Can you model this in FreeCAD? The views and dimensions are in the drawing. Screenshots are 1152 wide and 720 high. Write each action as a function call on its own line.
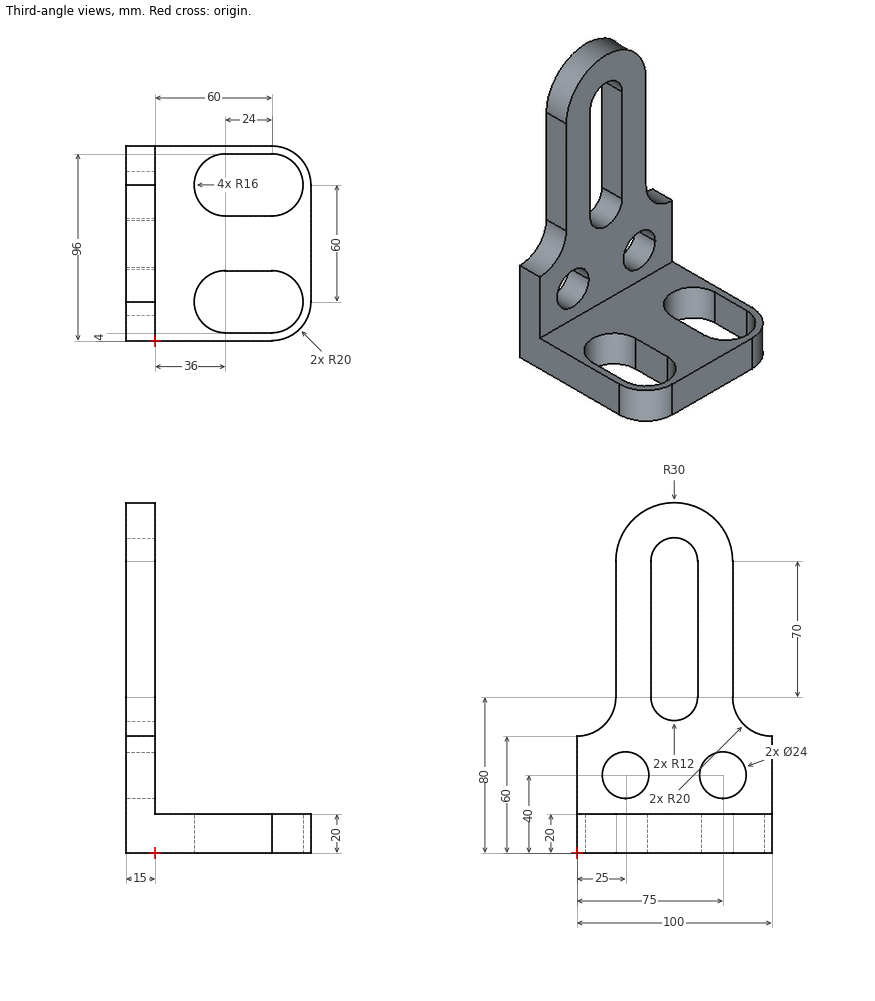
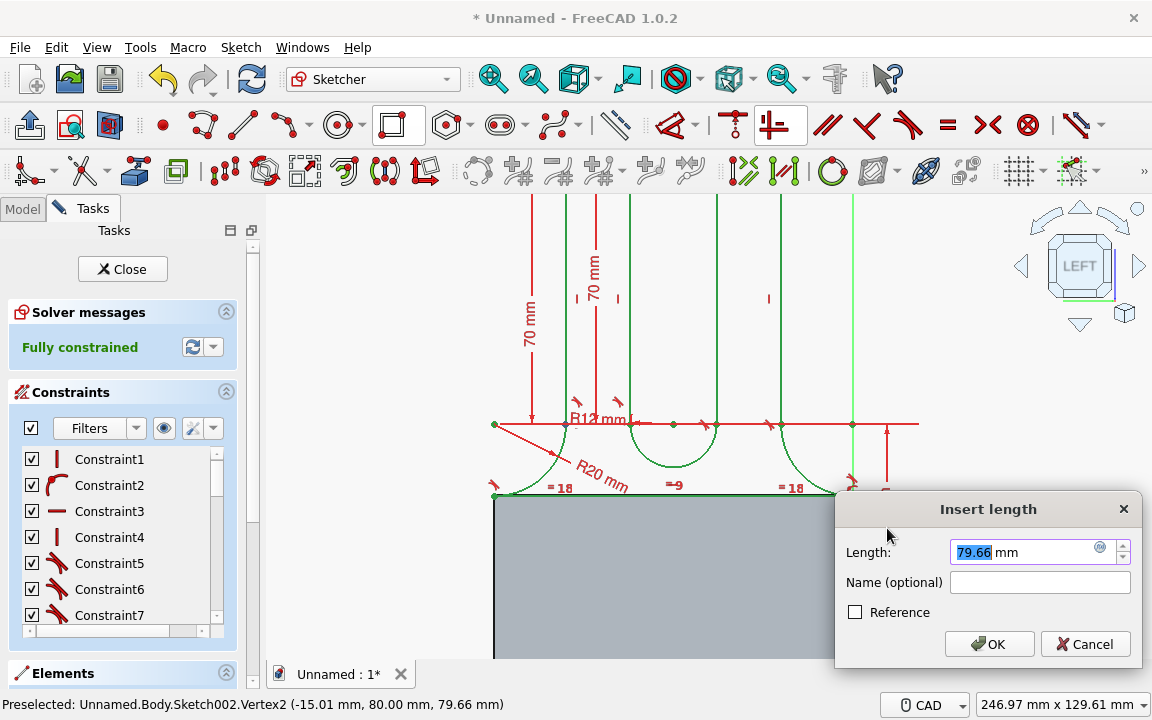
text(80)
key(Return)
key(Escape)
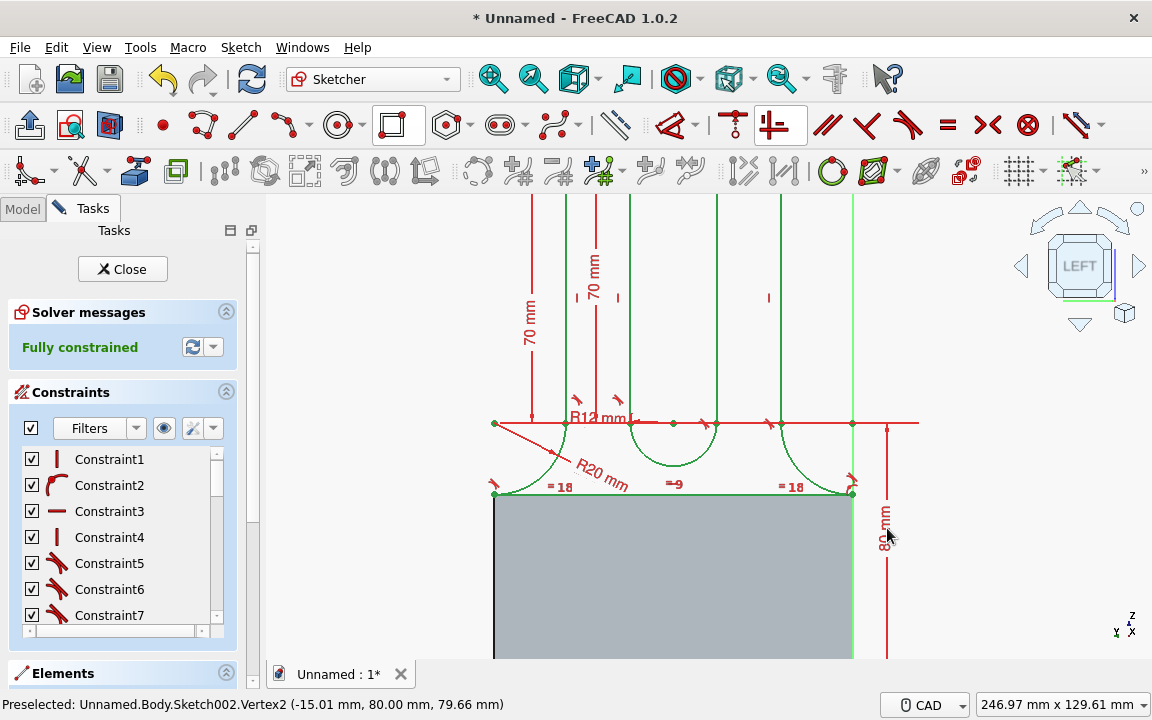
click(123, 269)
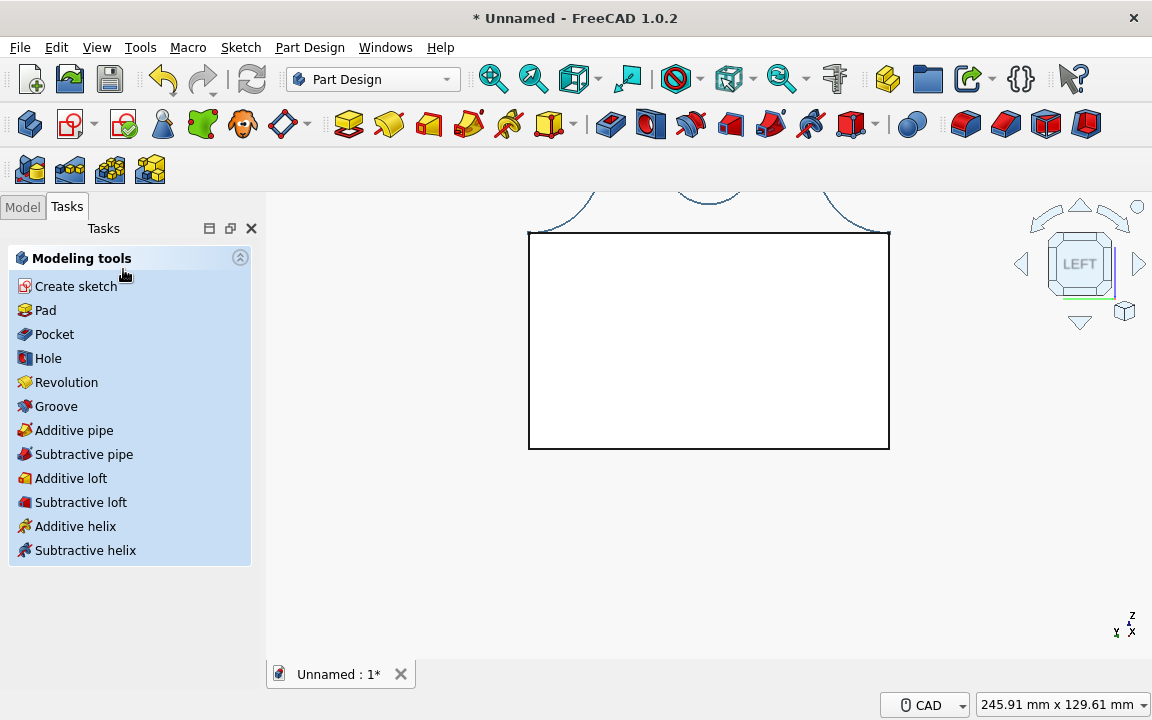
click(350, 124)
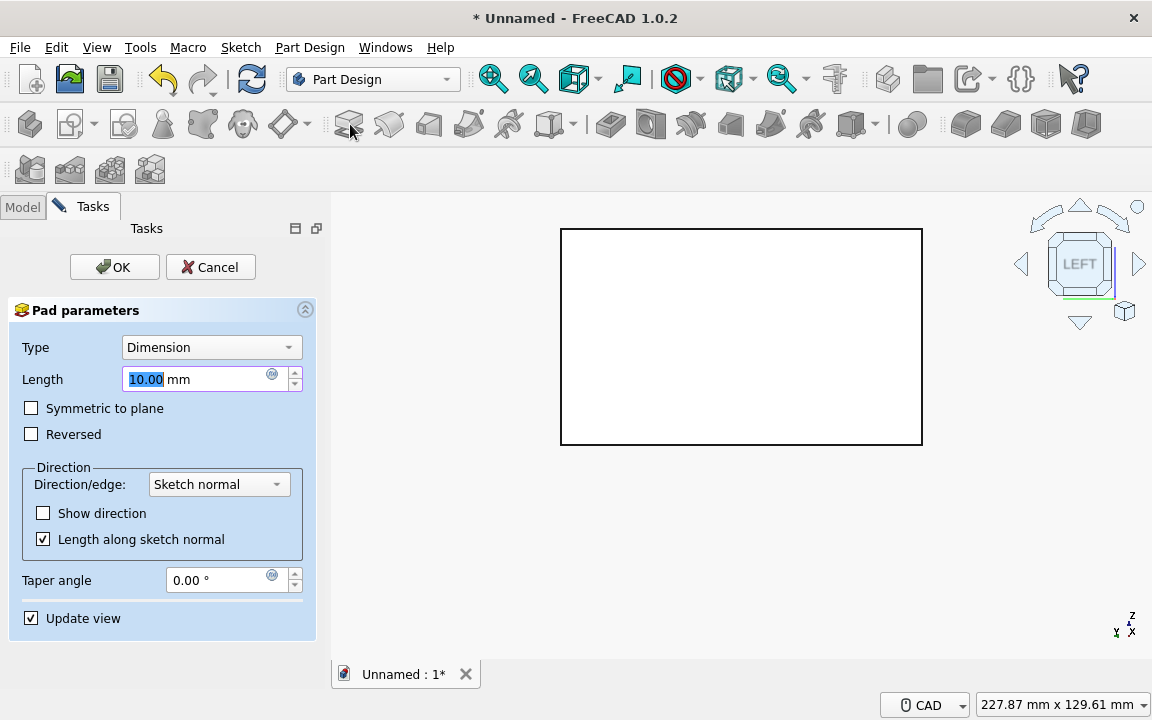
text(15)
key(Tab)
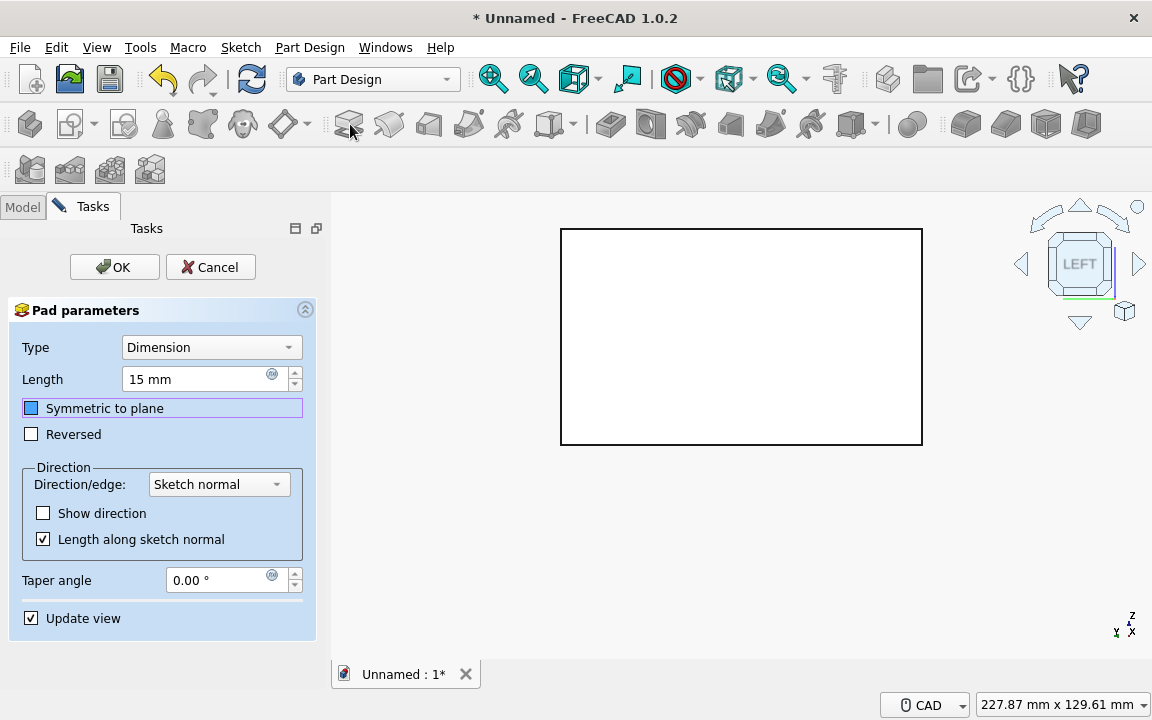
click(30, 434)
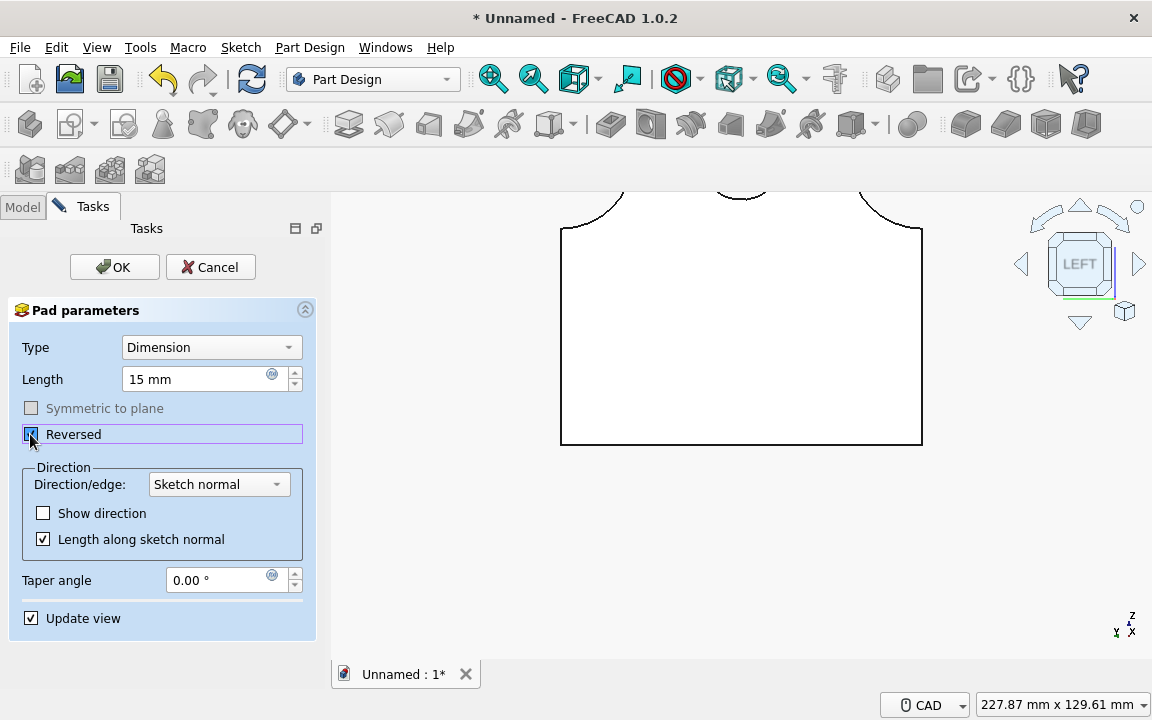
click(115, 267)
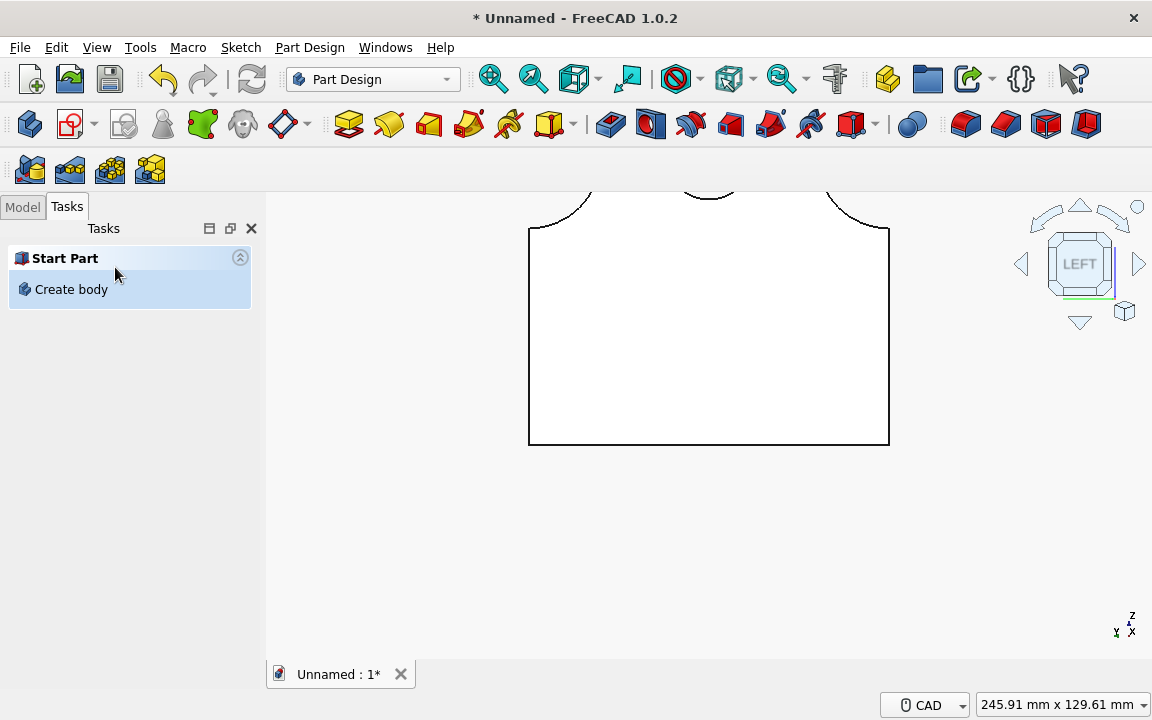
key(v)
key(f)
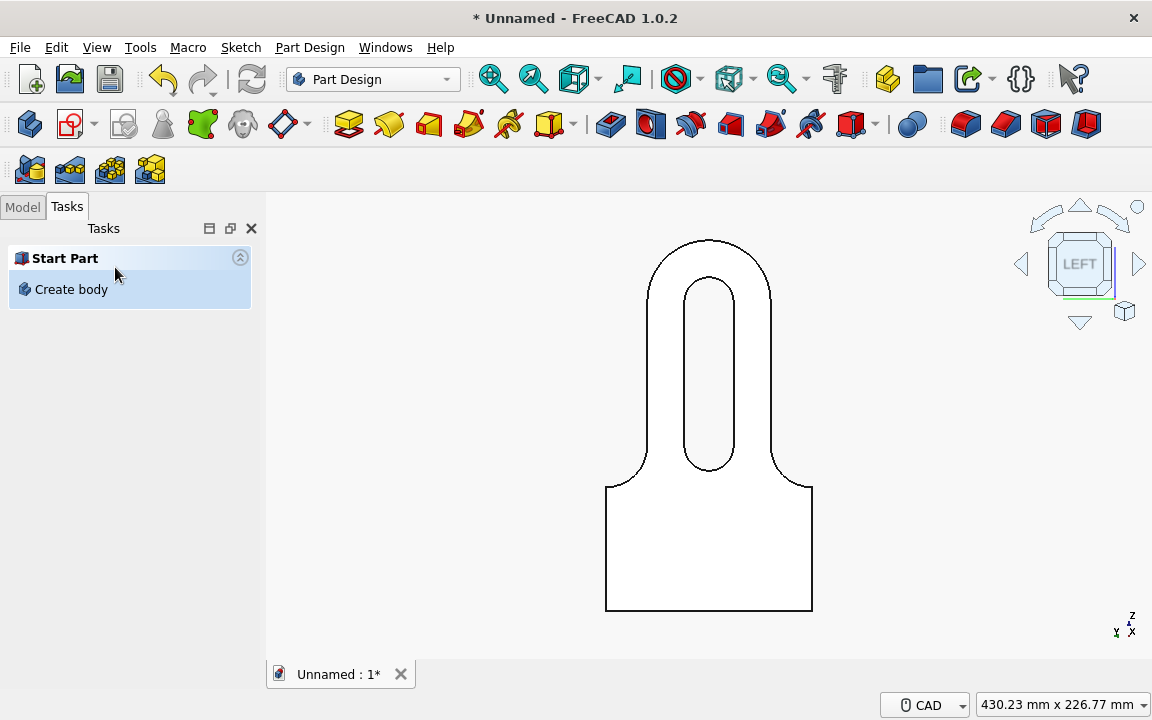
click(70, 124)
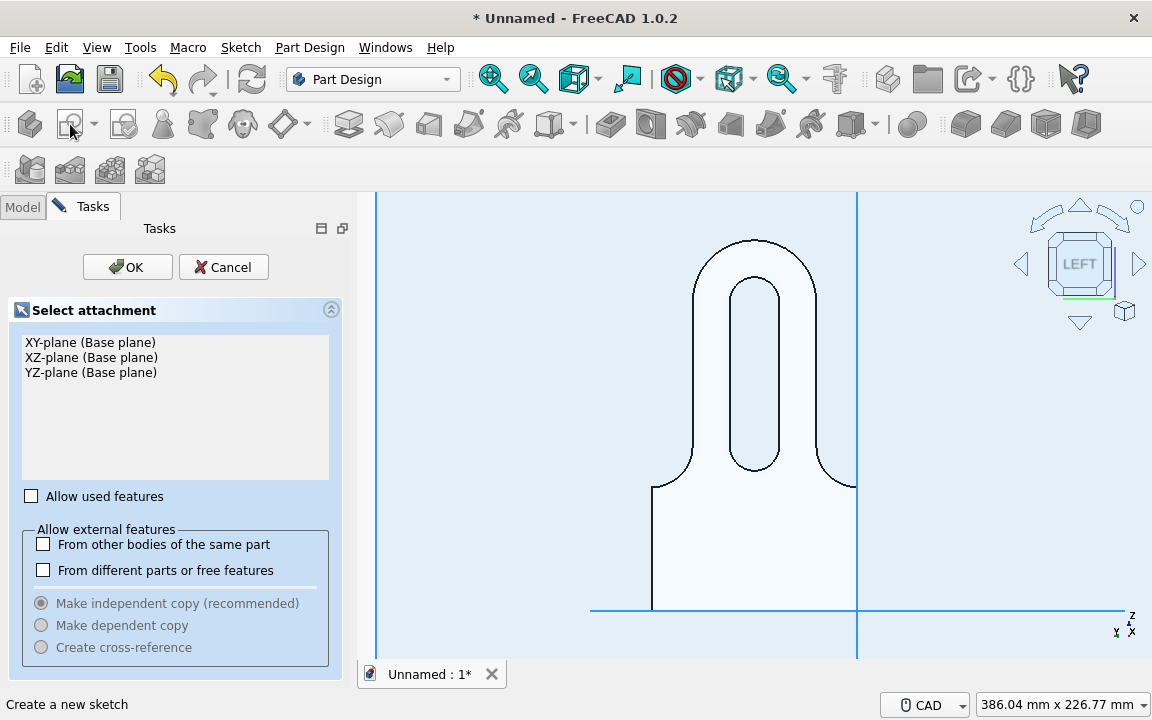
click(82, 372)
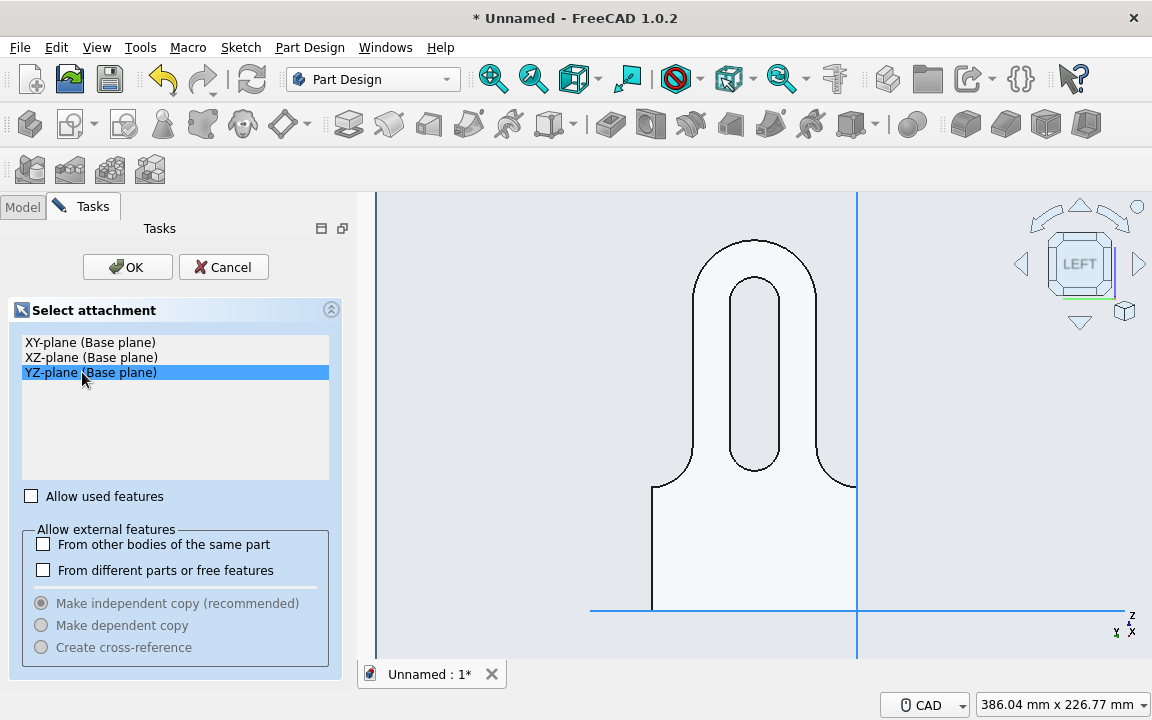
click(128, 267)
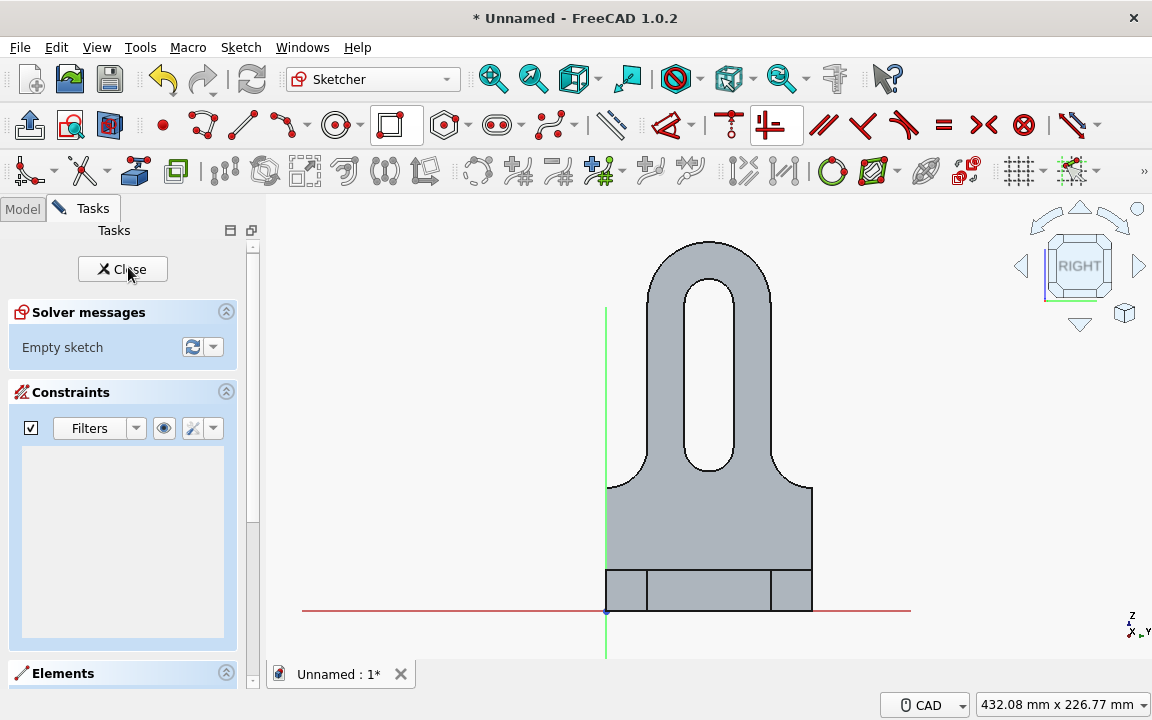
click(110, 126)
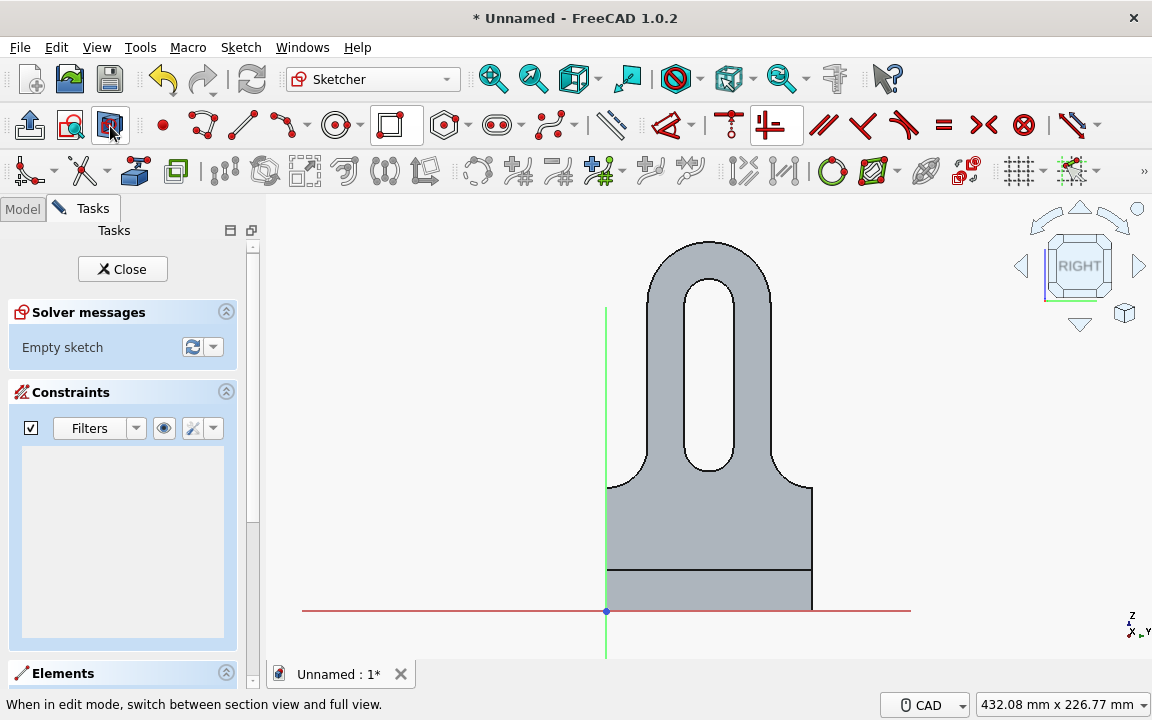
scroll(728, 631, up, 5)